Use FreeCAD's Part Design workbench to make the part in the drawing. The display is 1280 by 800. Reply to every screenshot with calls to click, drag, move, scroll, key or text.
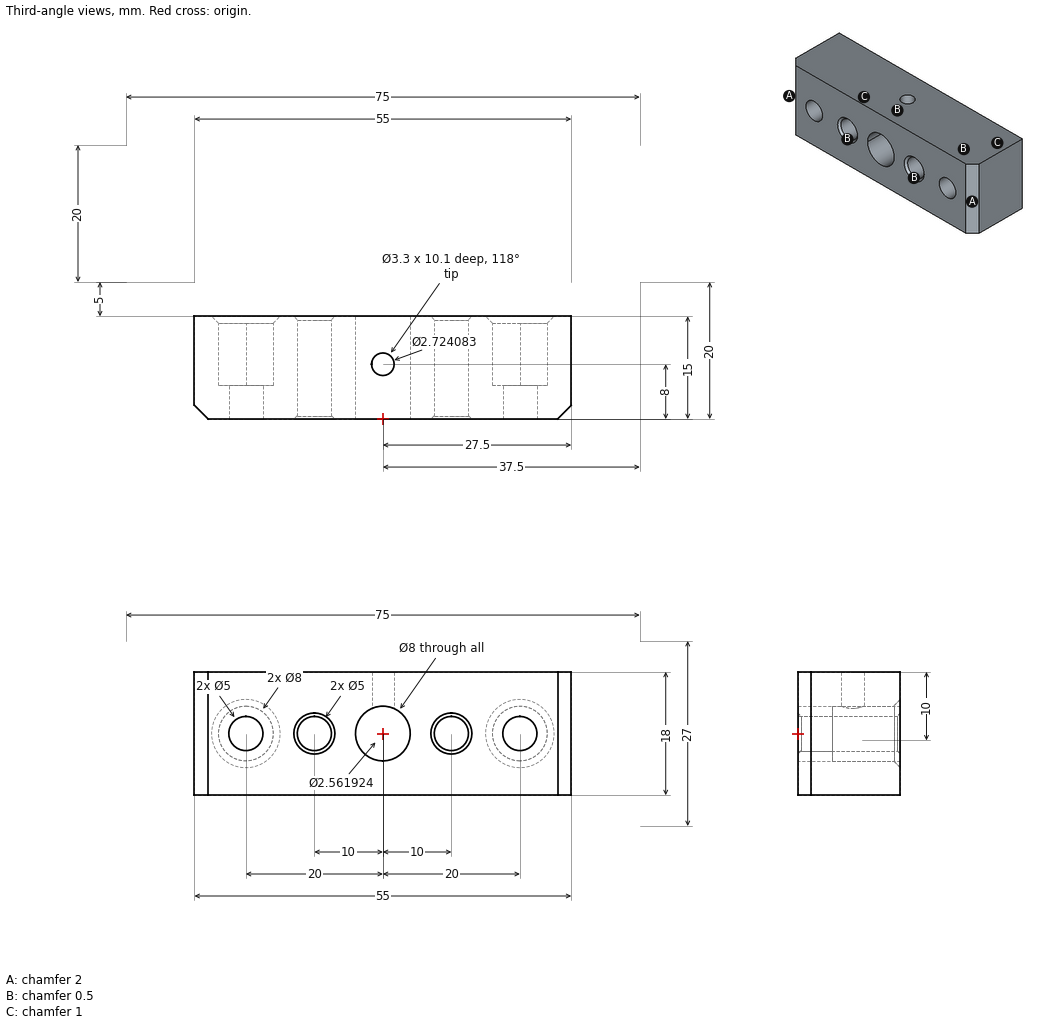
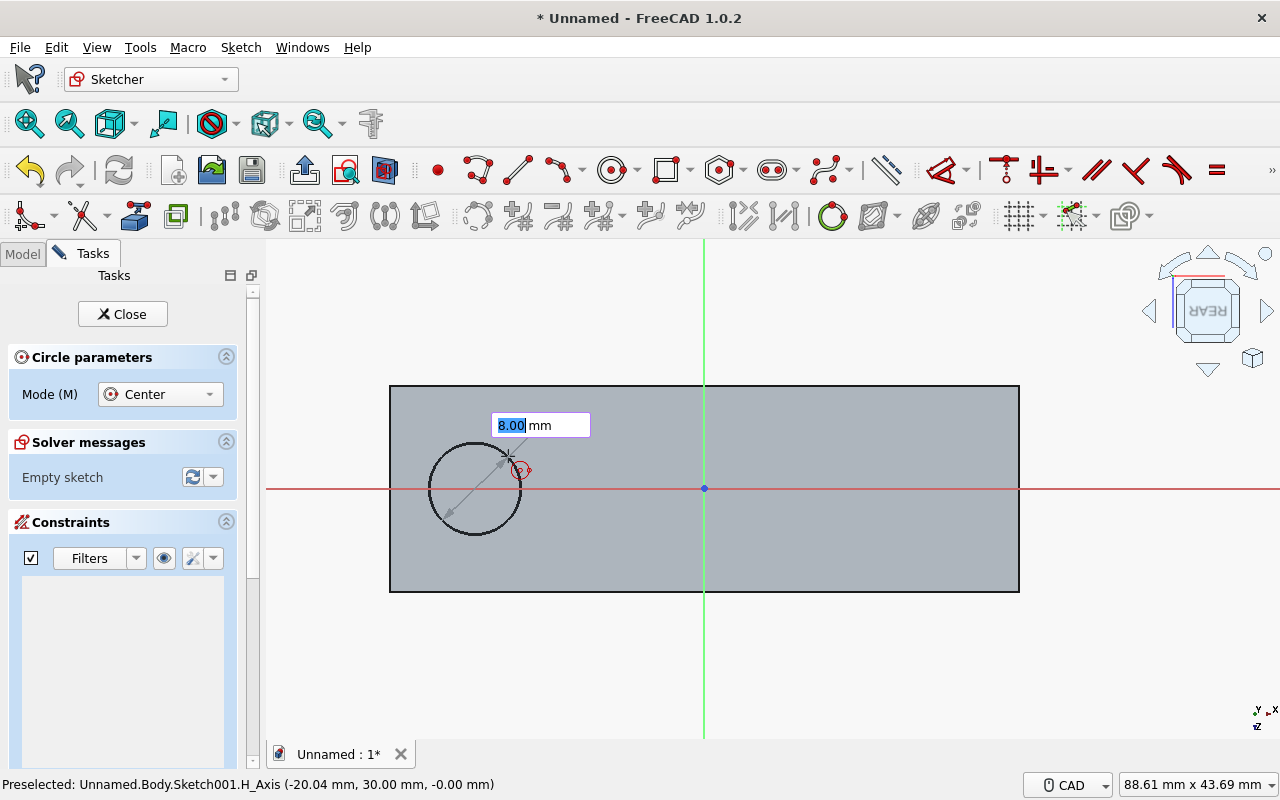
text(8)
key(Return)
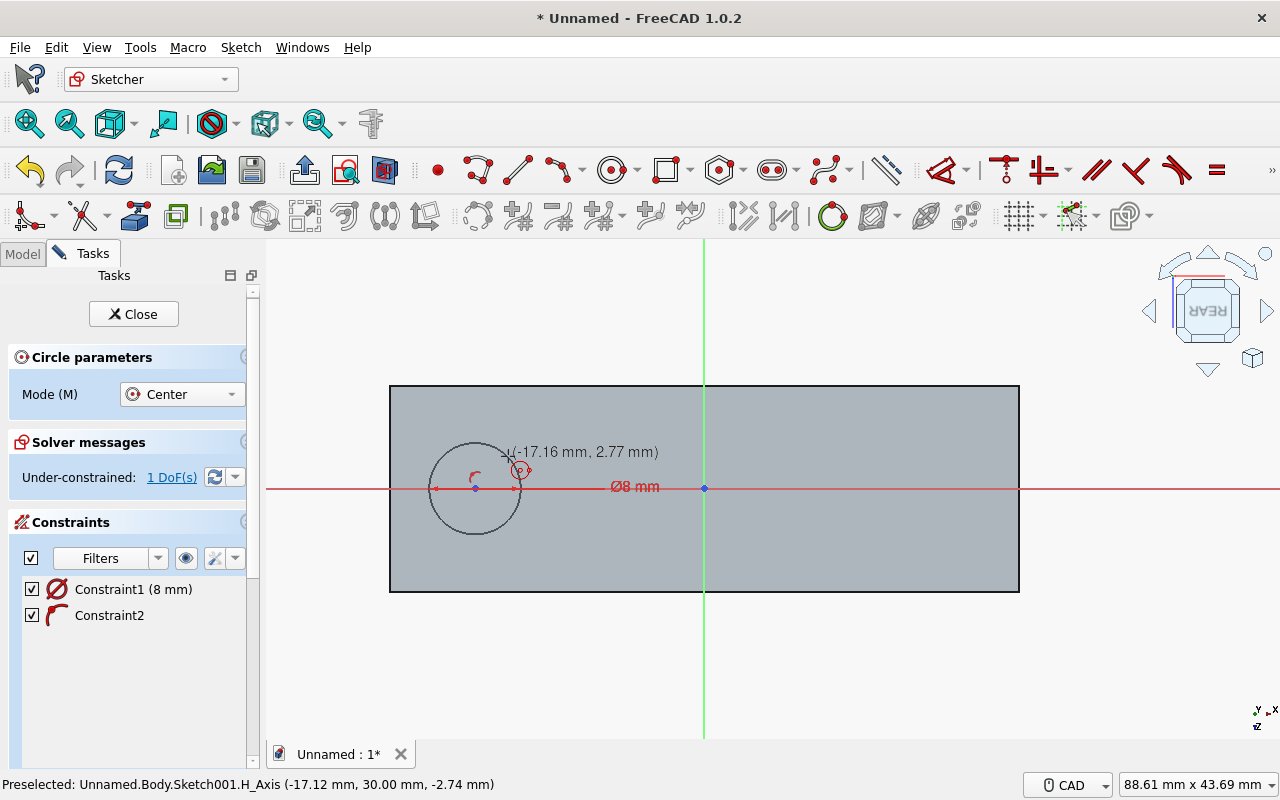
click(933, 489)
move(966, 456)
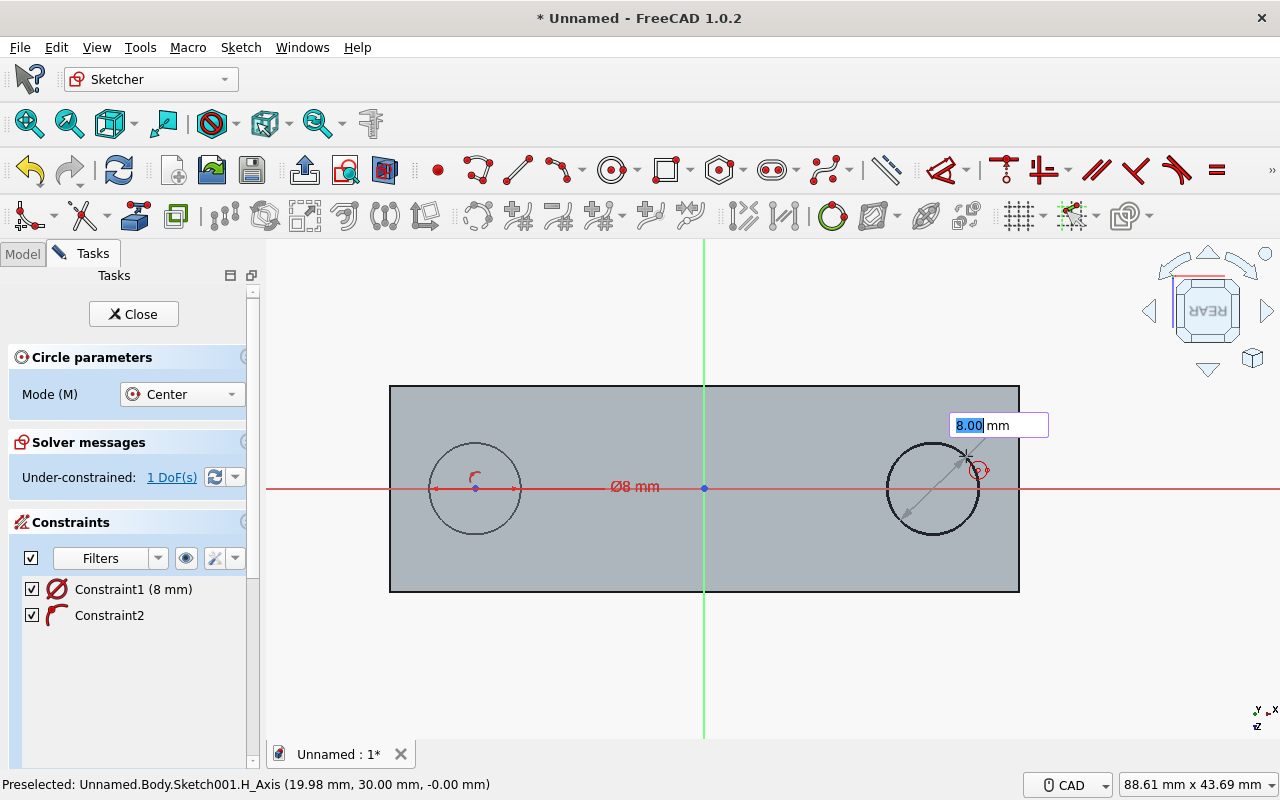
text(8)
key(Return)
key(Escape)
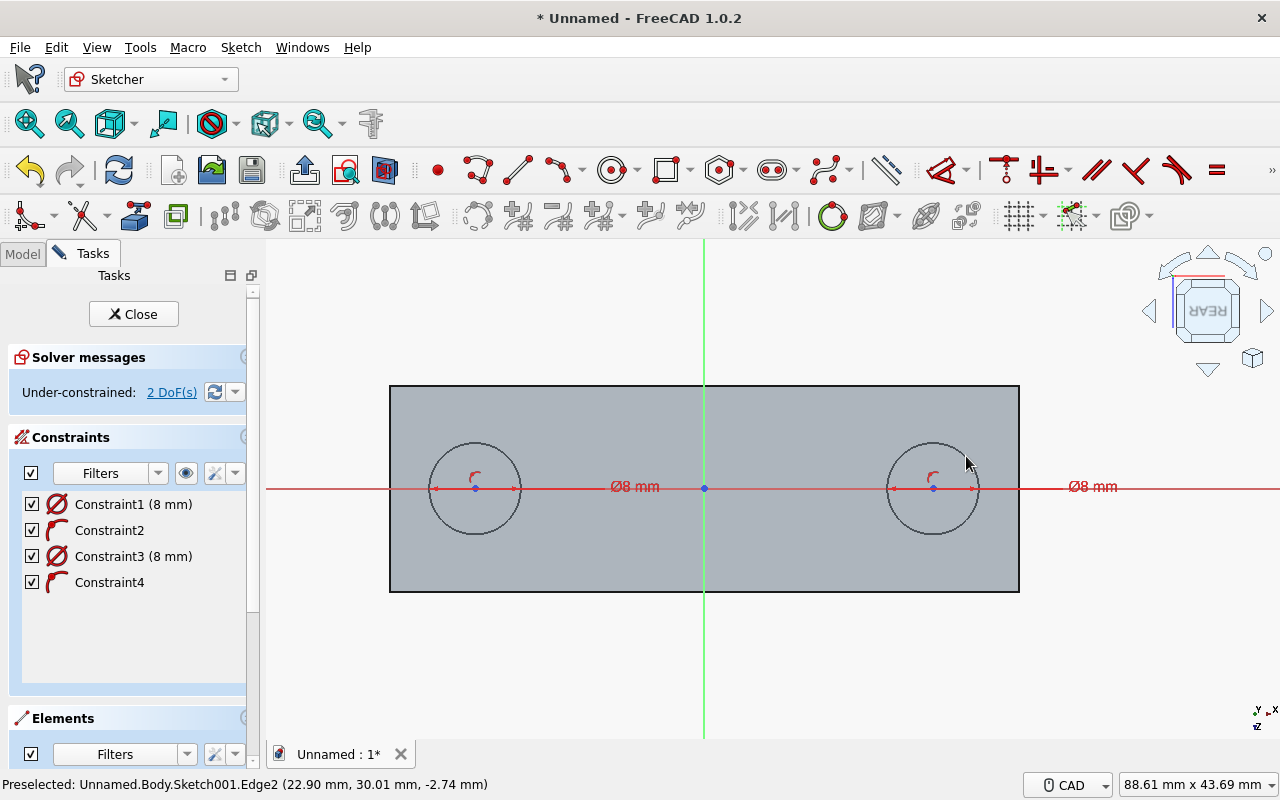
click(475, 489)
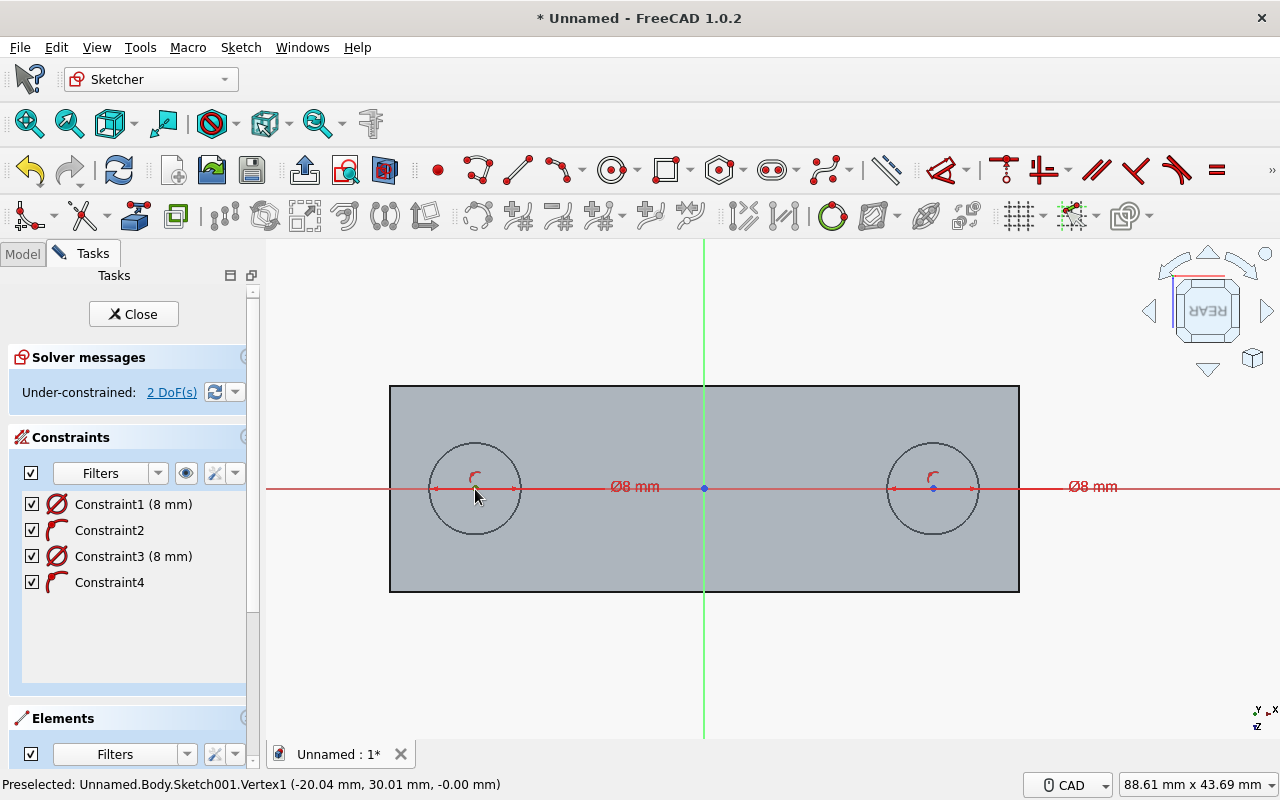
key(l)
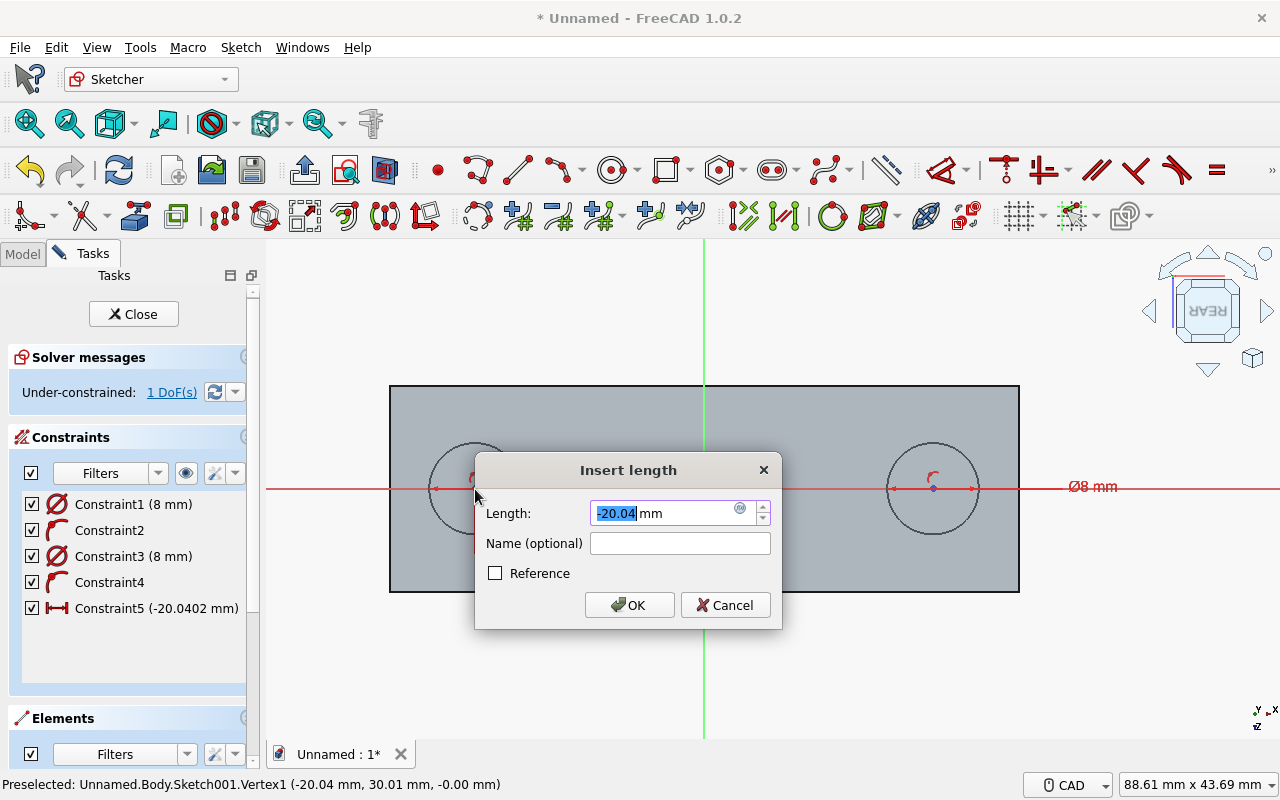
text(-20)
key(Return)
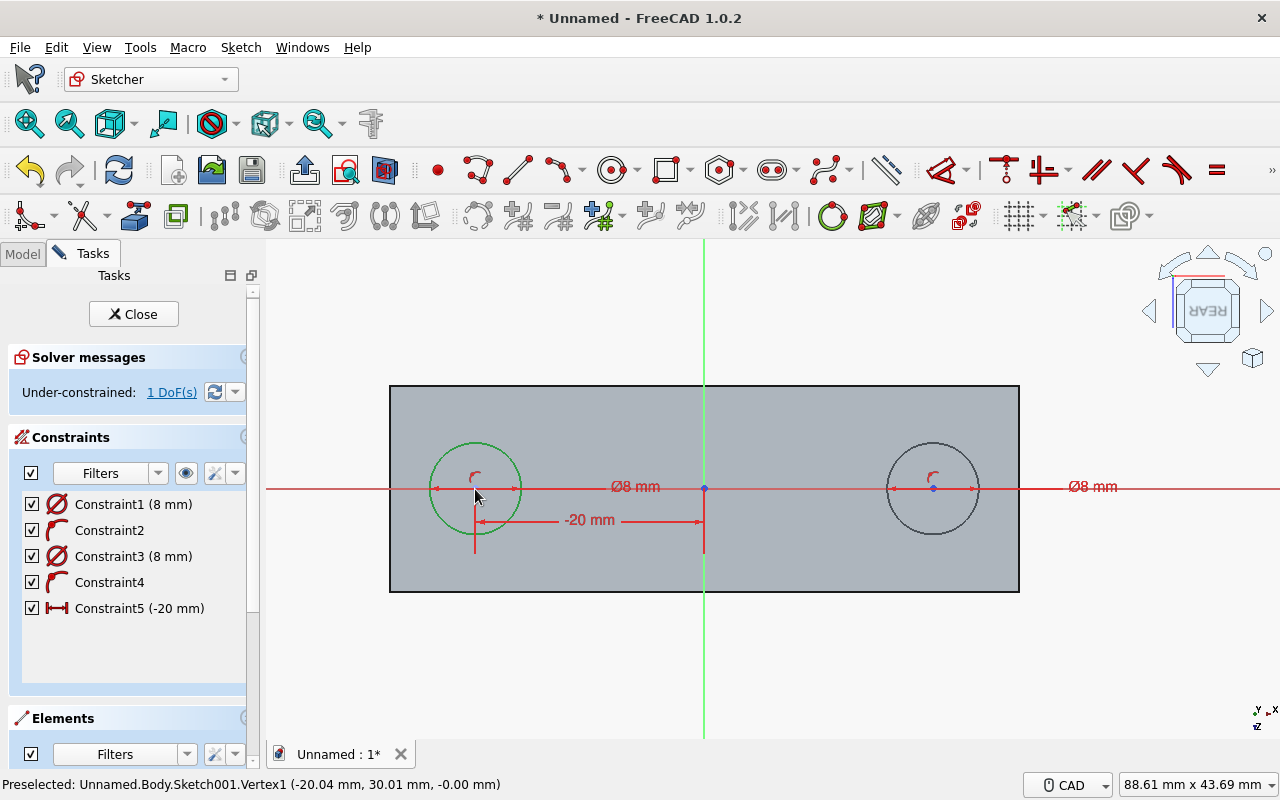
click(933, 489)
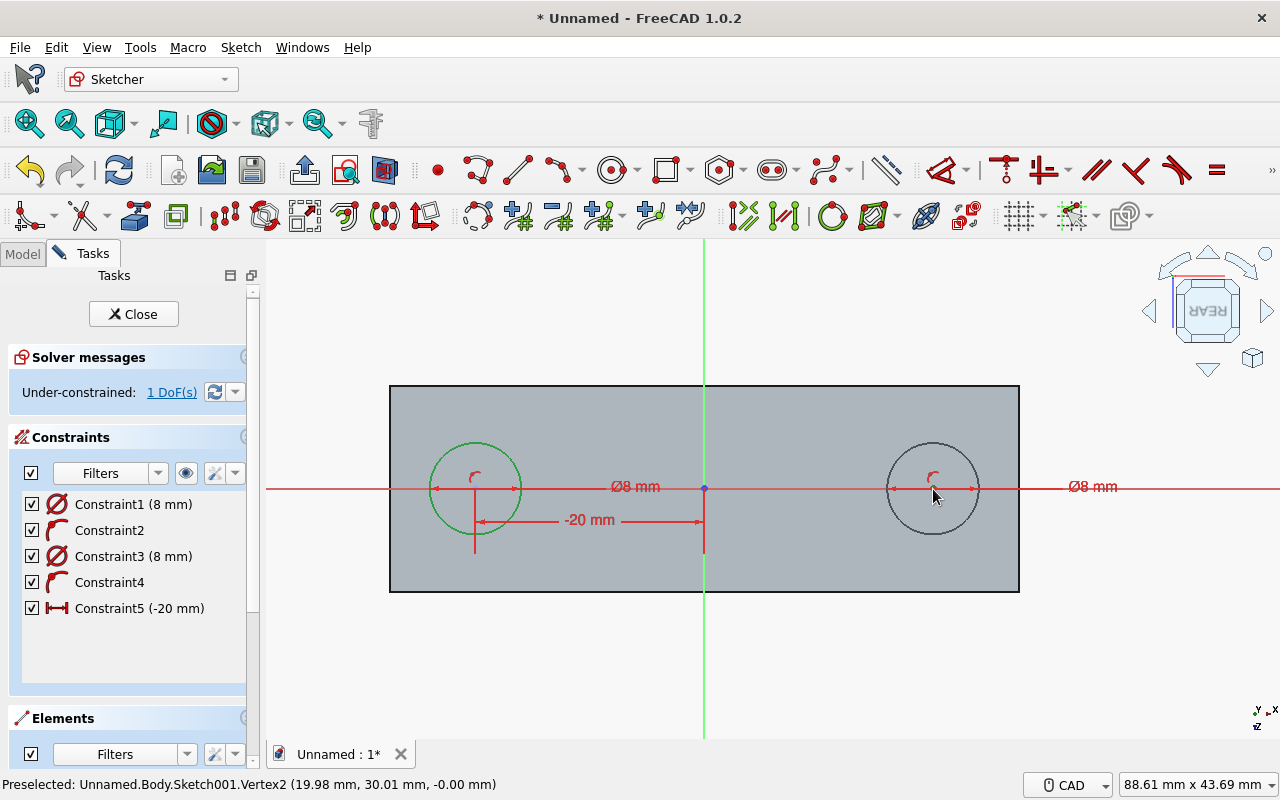
click(968, 170)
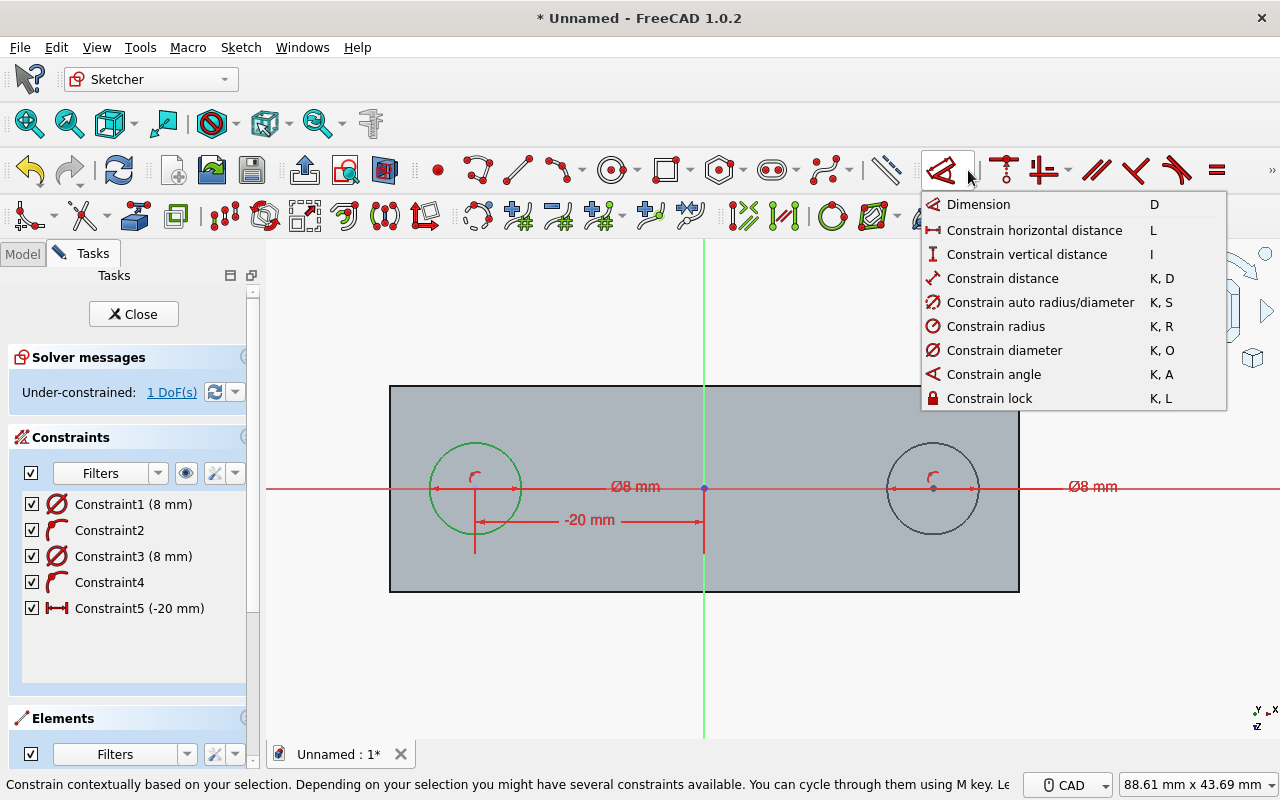
click(1074, 230)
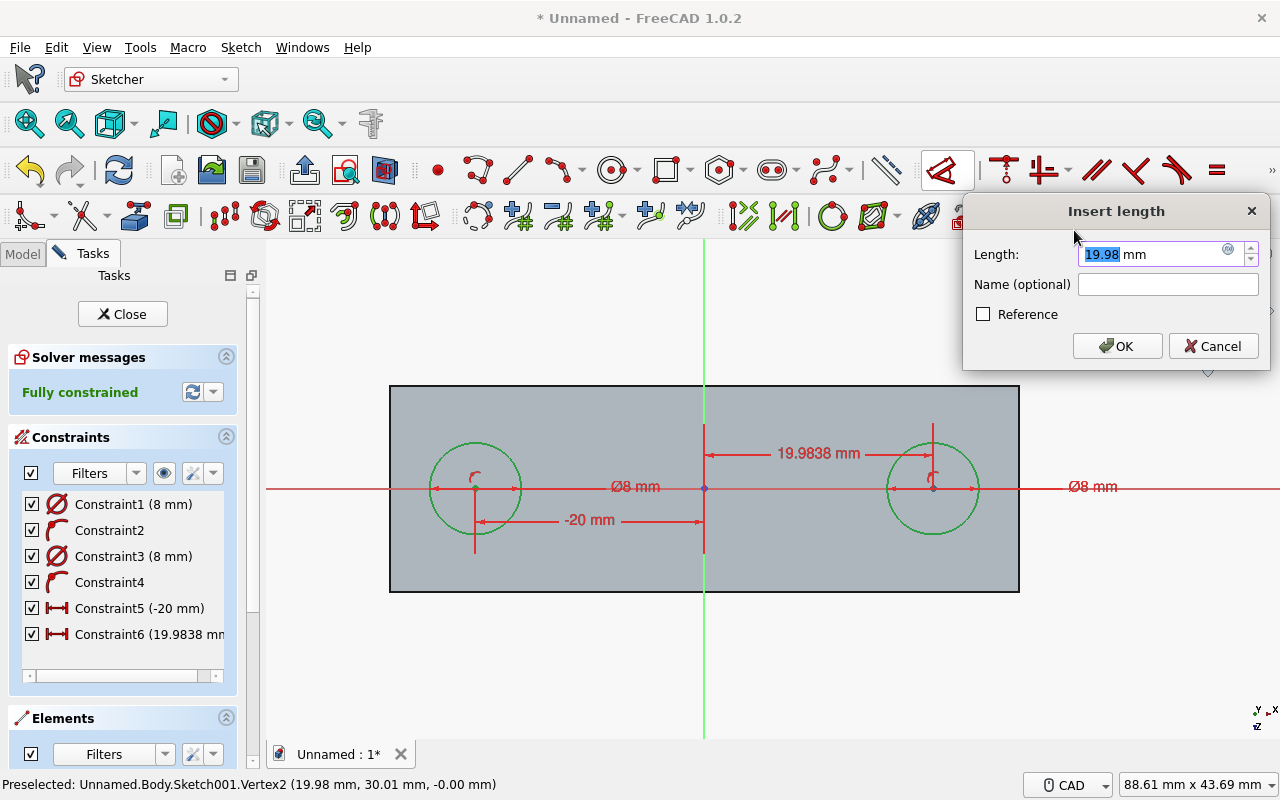
text(20)
key(Return)